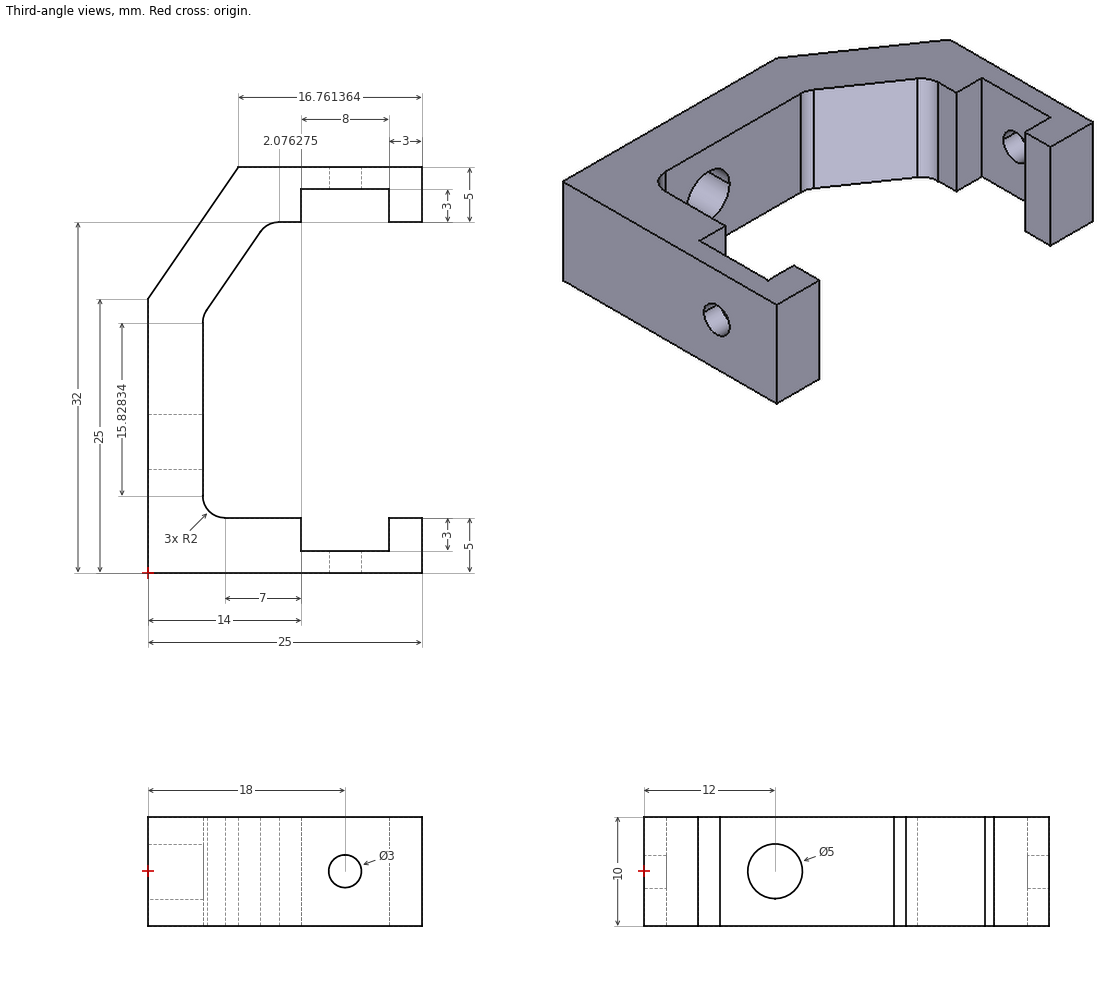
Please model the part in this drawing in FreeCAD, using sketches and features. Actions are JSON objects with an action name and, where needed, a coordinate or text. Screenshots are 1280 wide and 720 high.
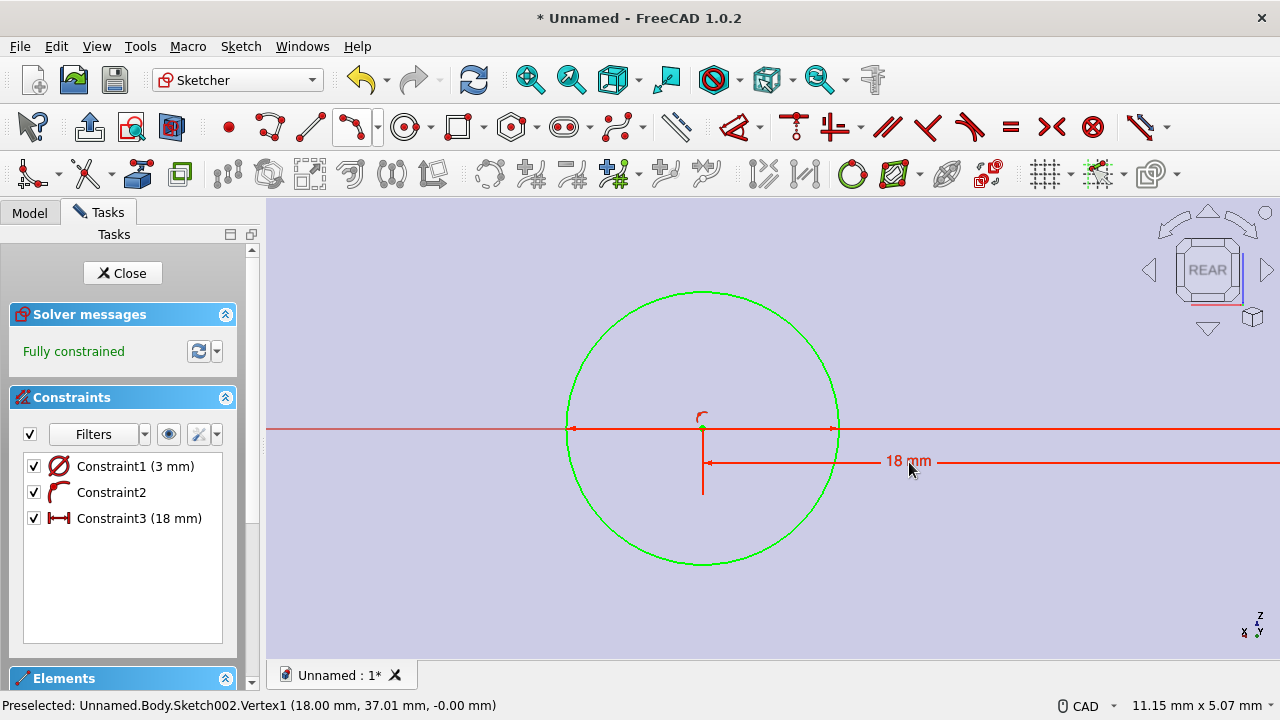
{"action": "left_click", "coordinate": [123, 273]}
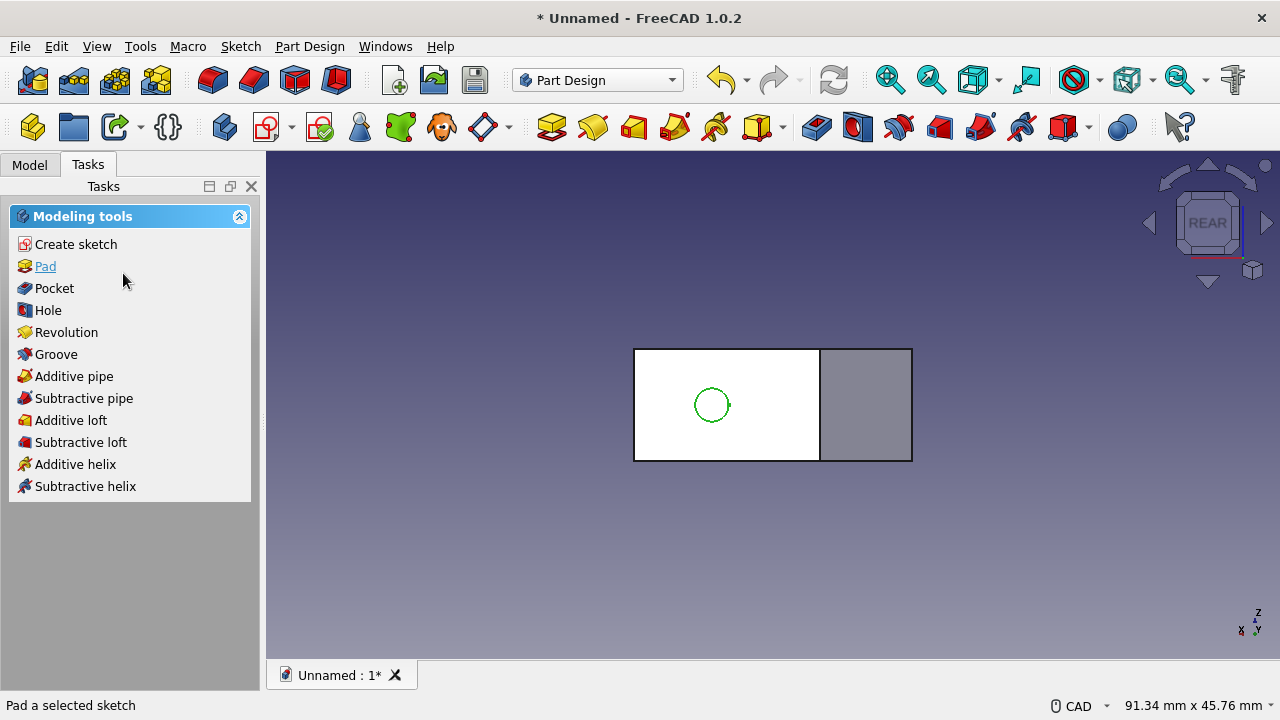
{"action": "left_click", "coordinate": [817, 128]}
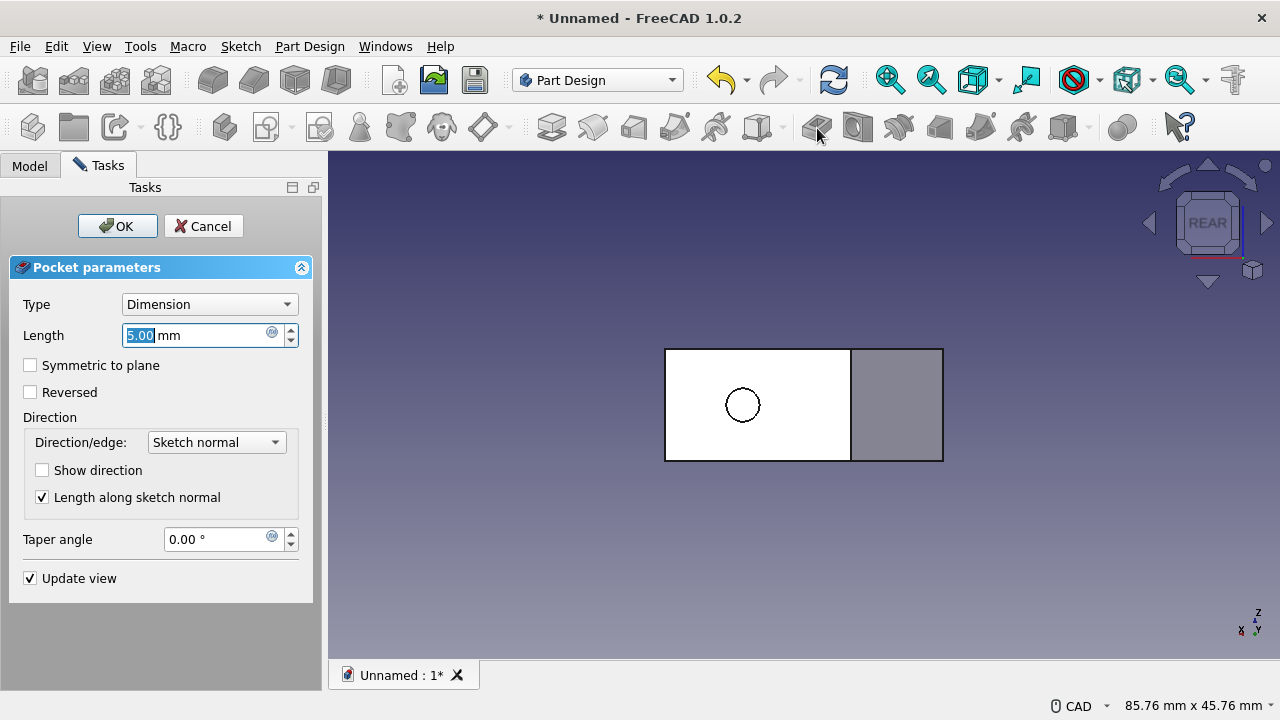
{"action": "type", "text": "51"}
{"action": "key", "text": "Tab"}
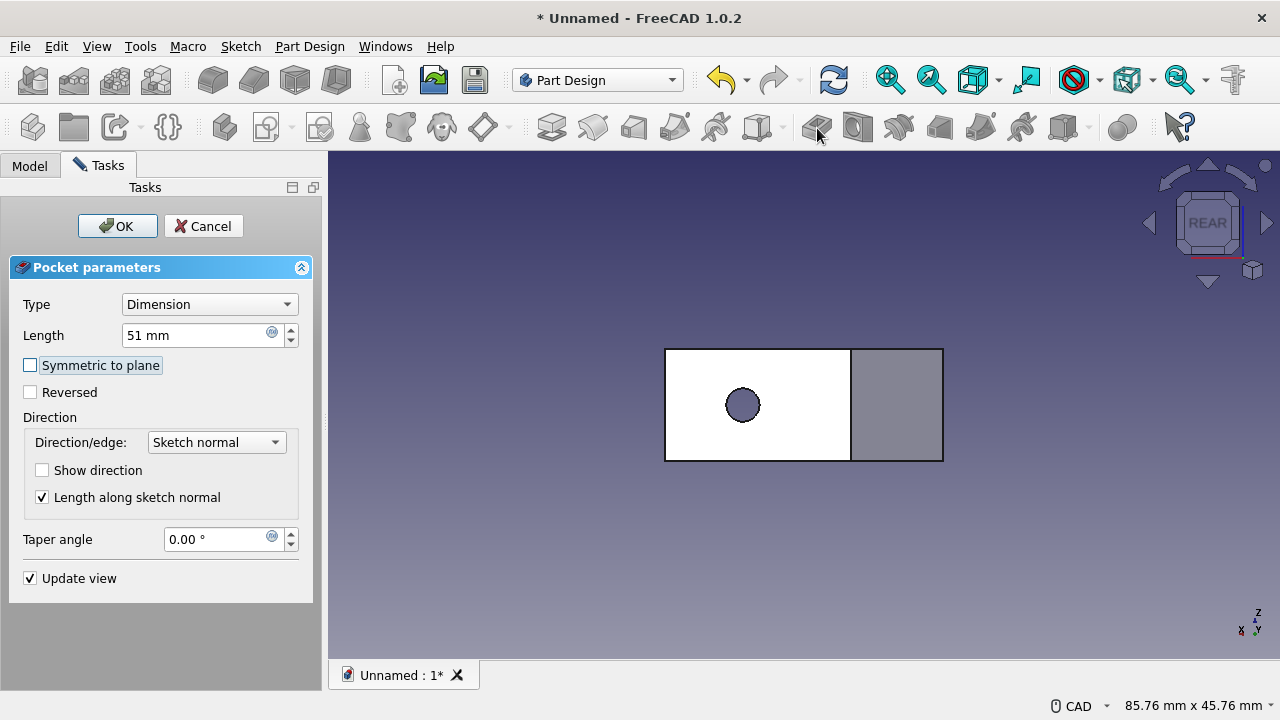
{"action": "left_click", "coordinate": [118, 226]}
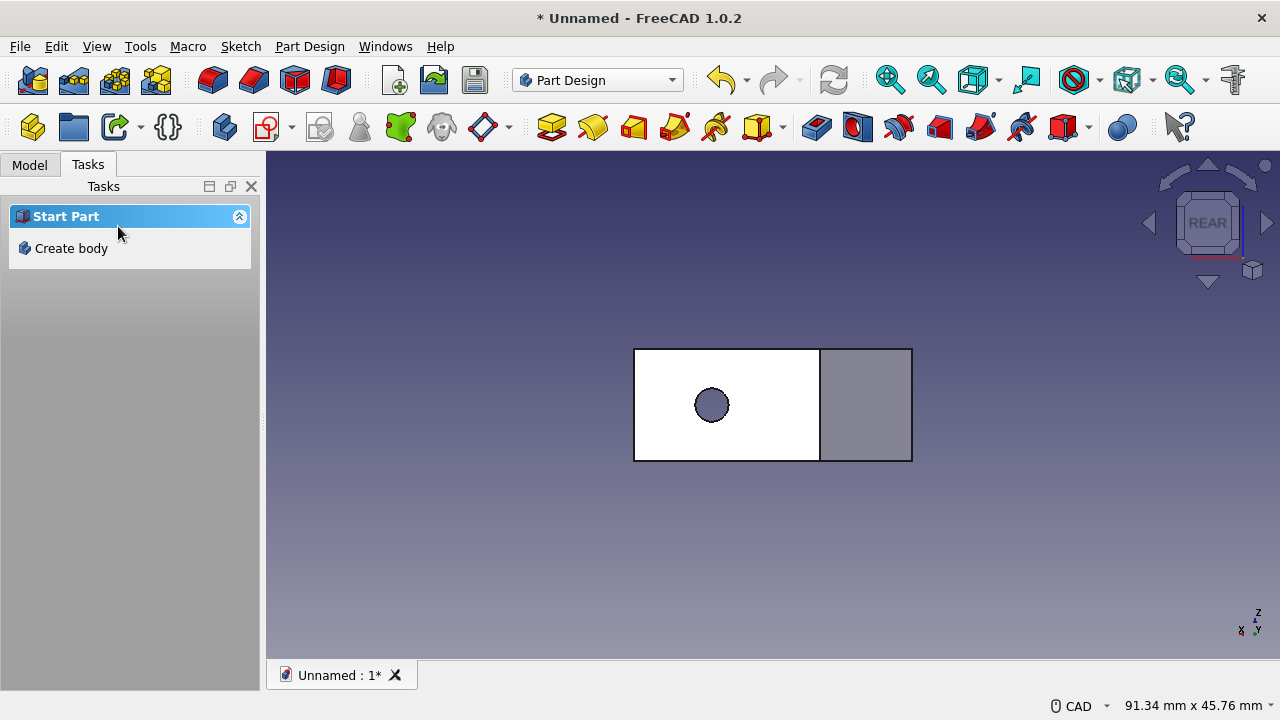
{"action": "key", "text": "0"}